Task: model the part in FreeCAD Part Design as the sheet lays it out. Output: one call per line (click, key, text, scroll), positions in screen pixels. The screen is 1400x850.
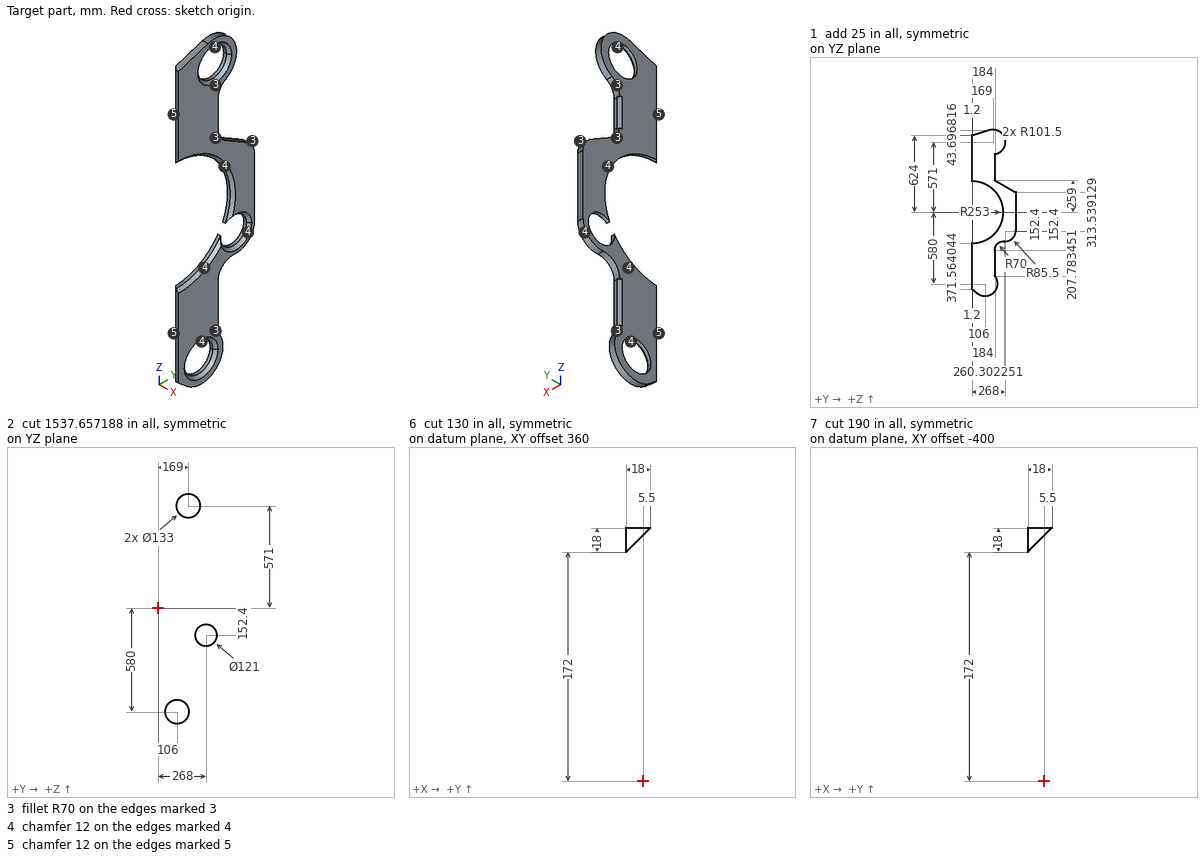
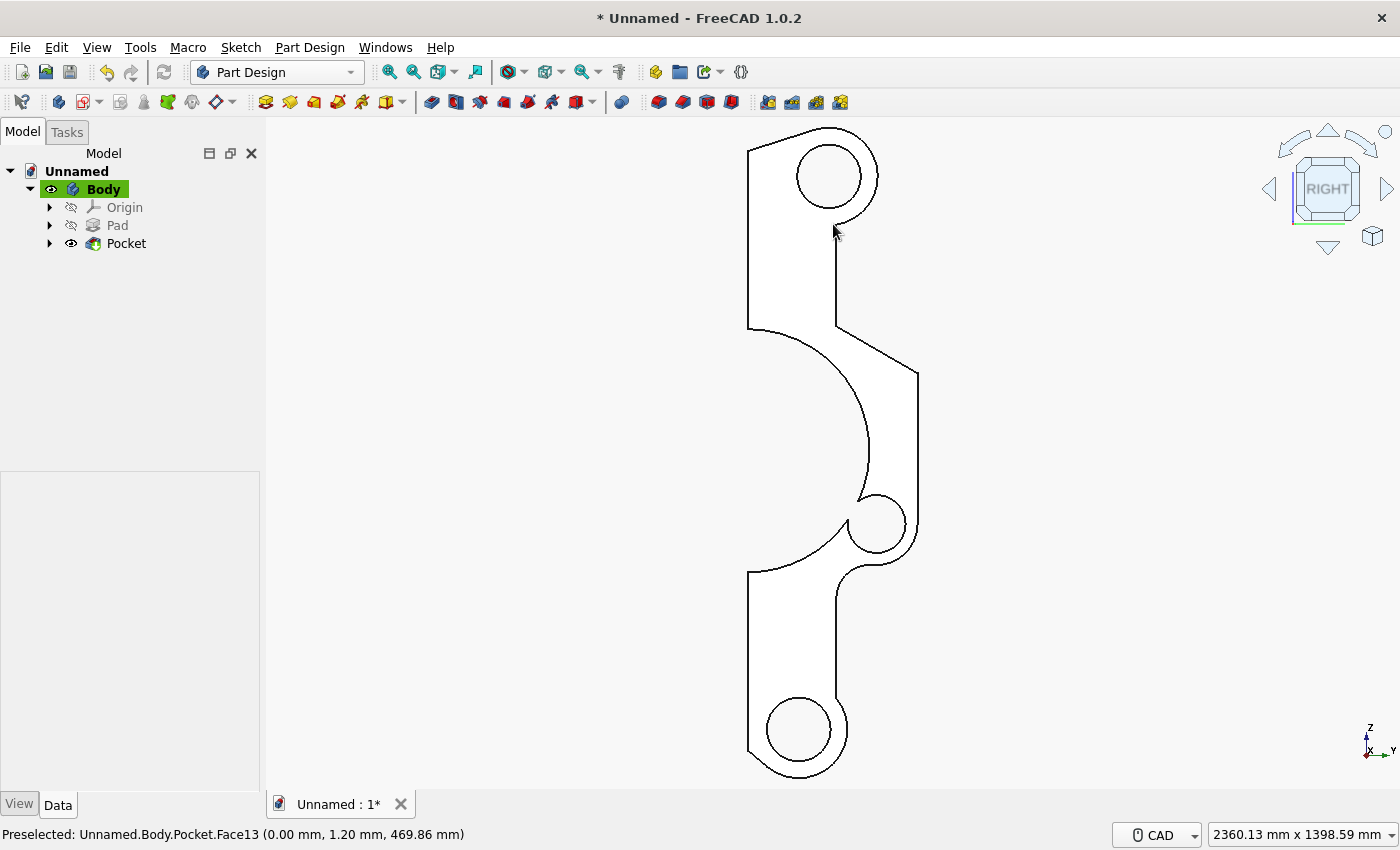
scroll(836, 224, up, 7)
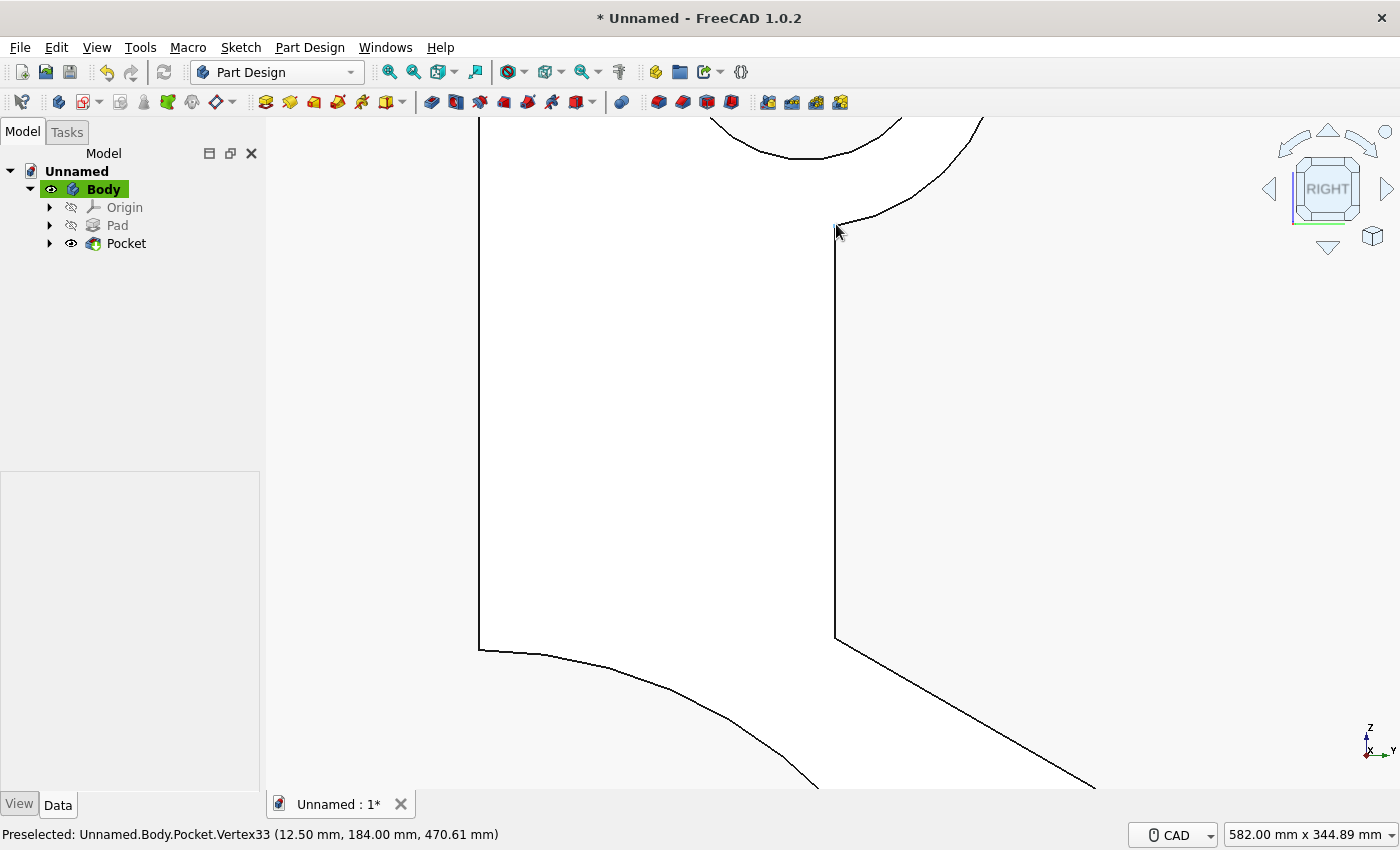
key(v)
key(f)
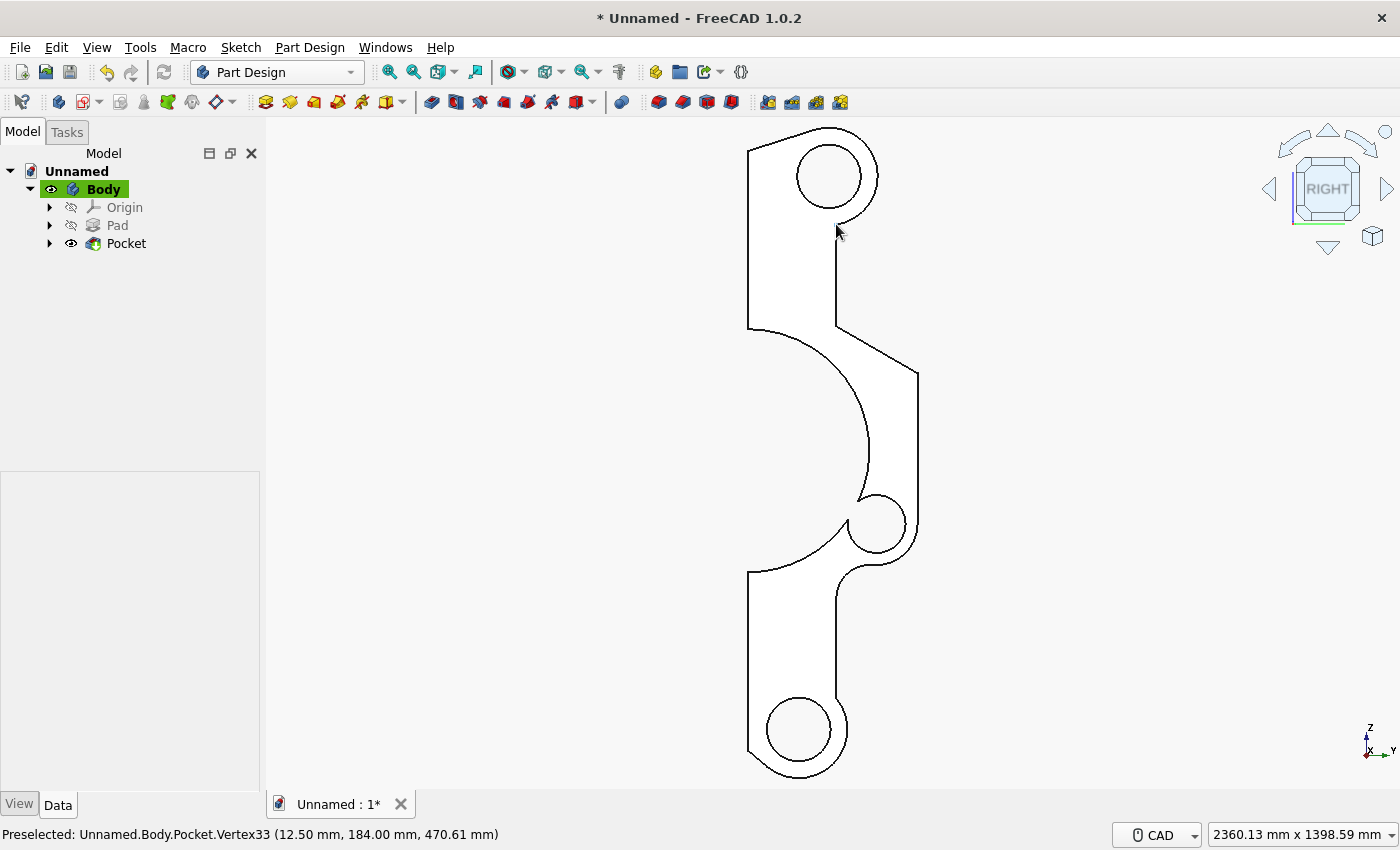
key(5)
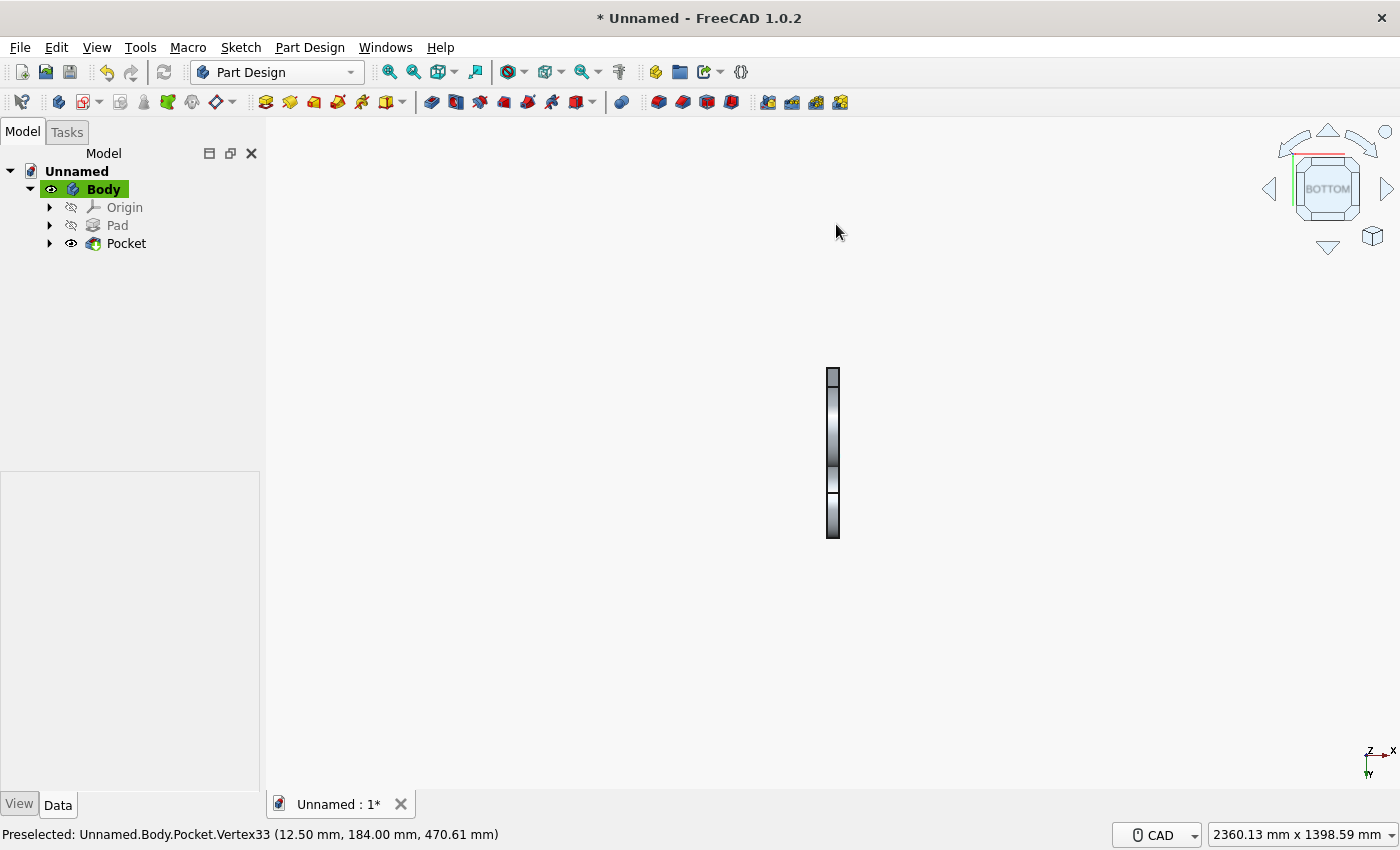
click(390, 72)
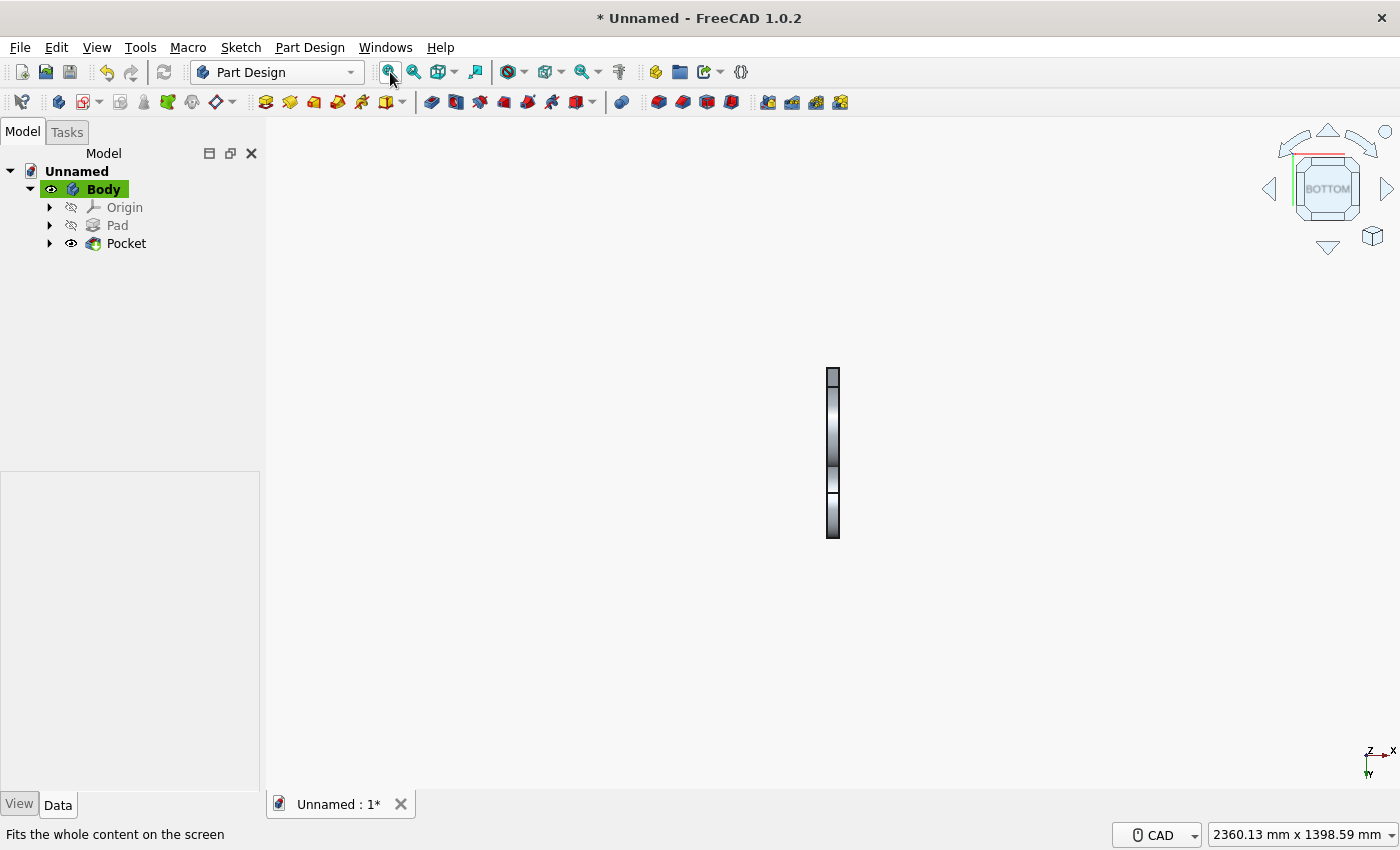
scroll(833, 455, up, 7)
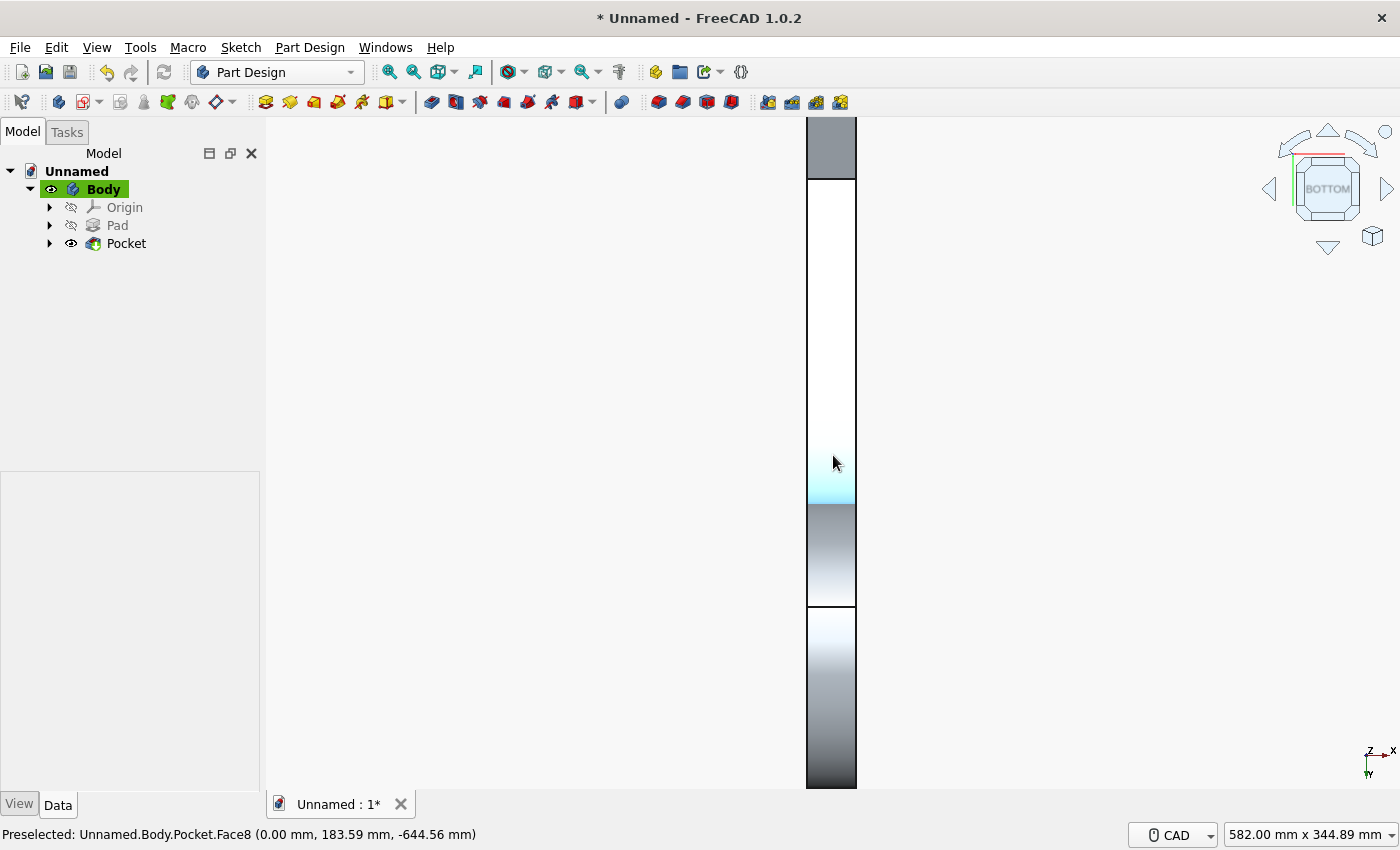
click(390, 72)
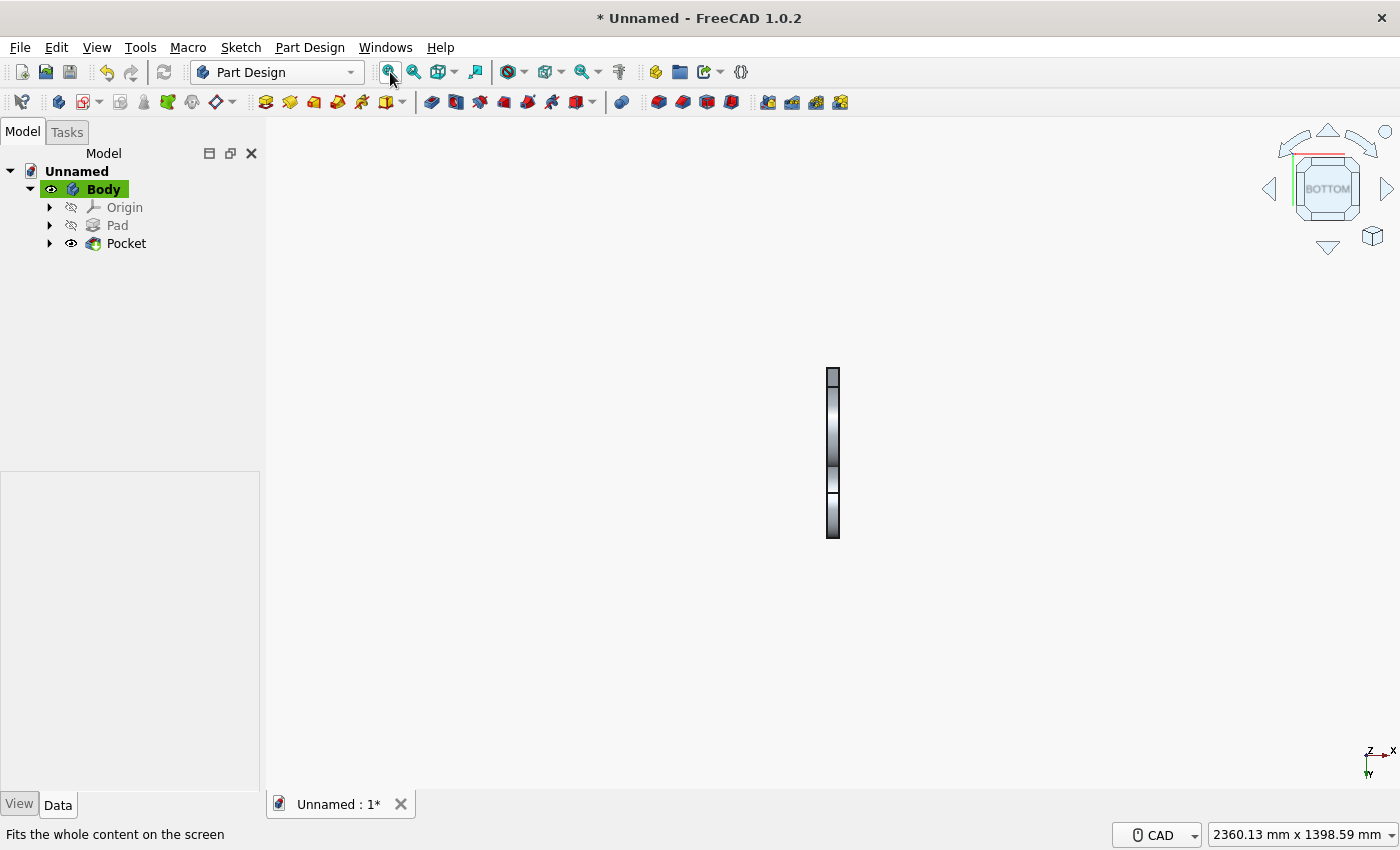
key(4)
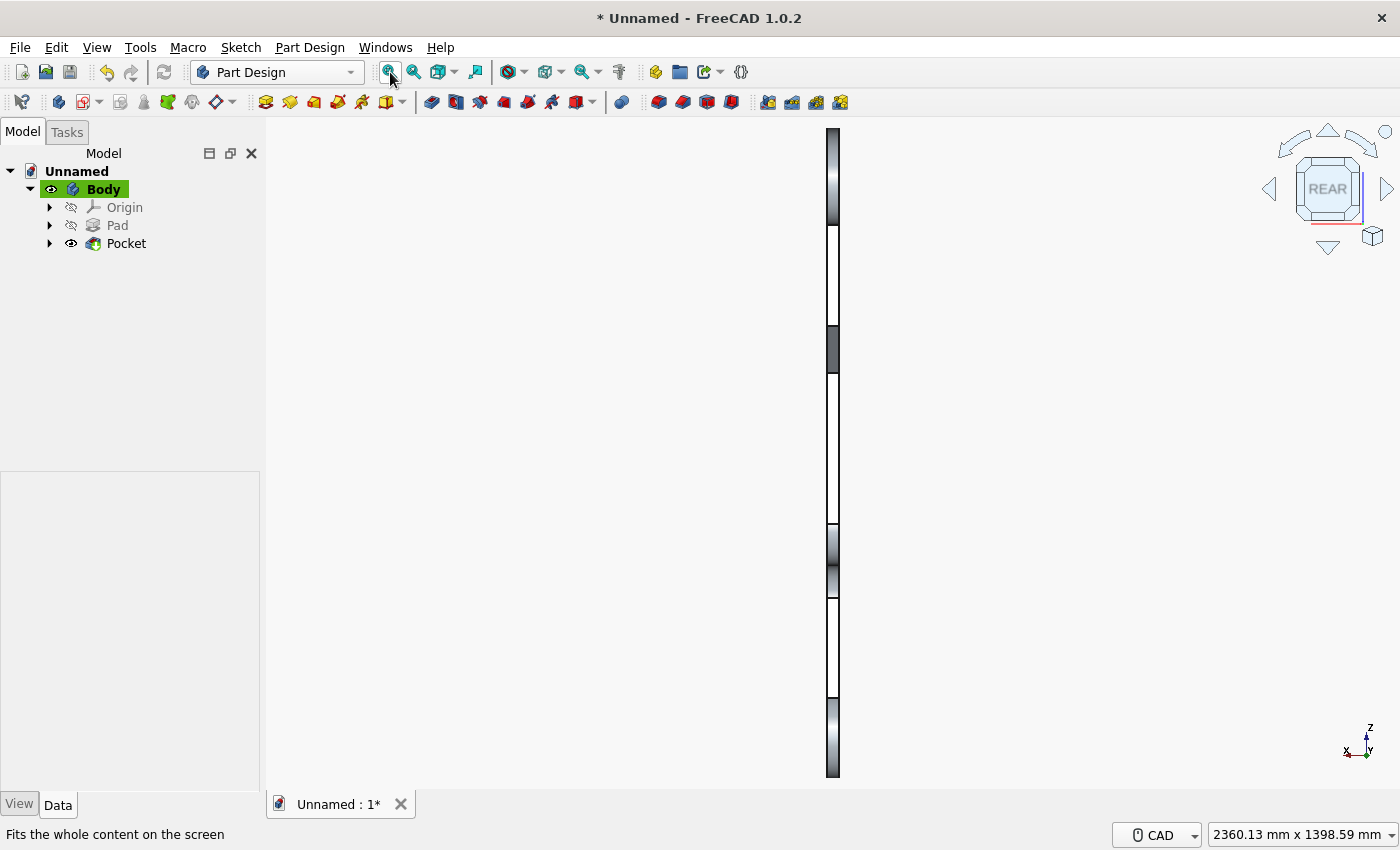
click(833, 372)